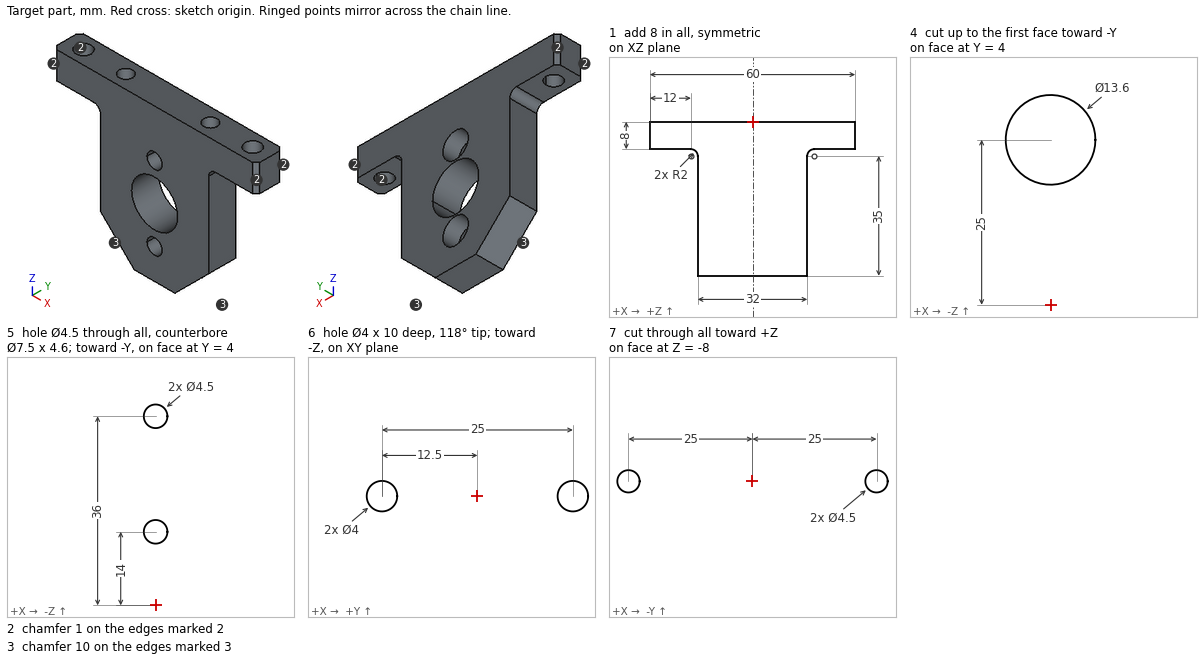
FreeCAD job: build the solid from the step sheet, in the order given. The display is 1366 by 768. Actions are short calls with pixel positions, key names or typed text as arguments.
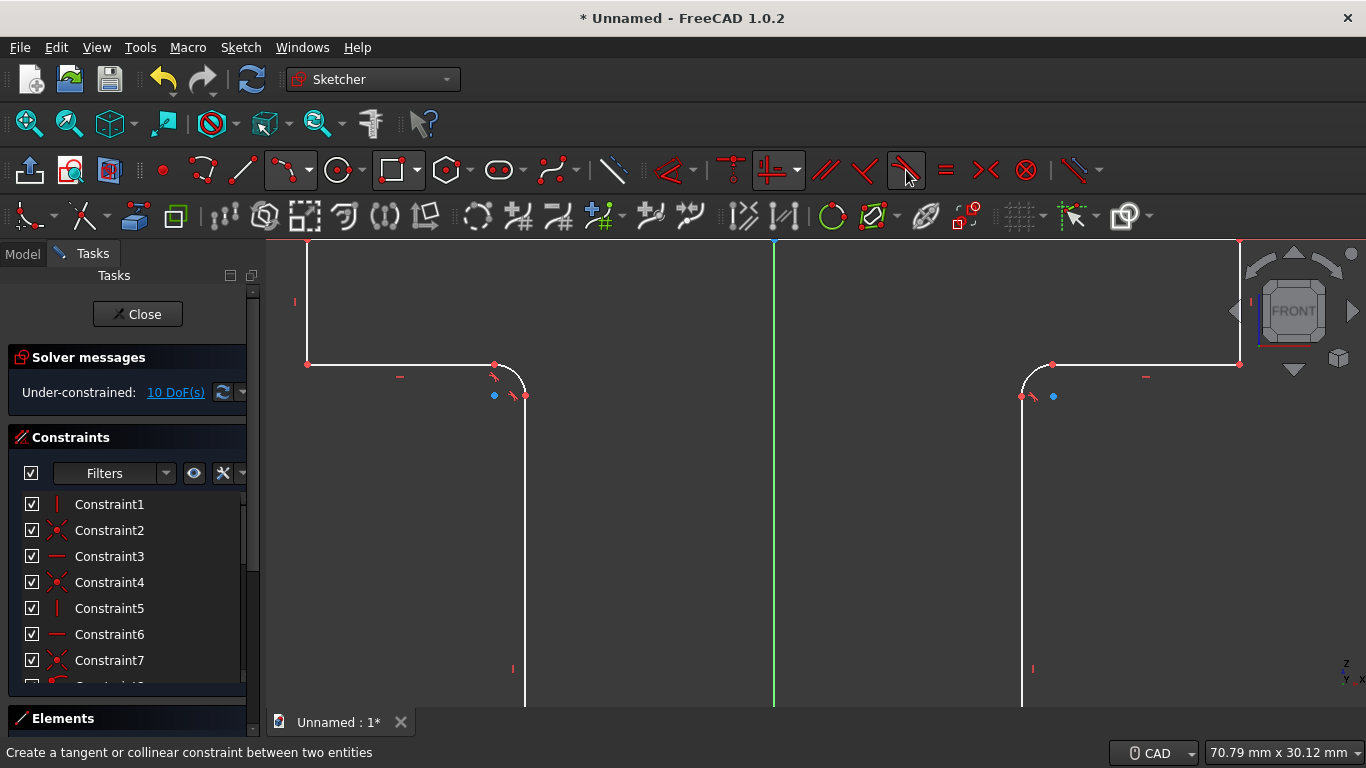
click(1184, 365)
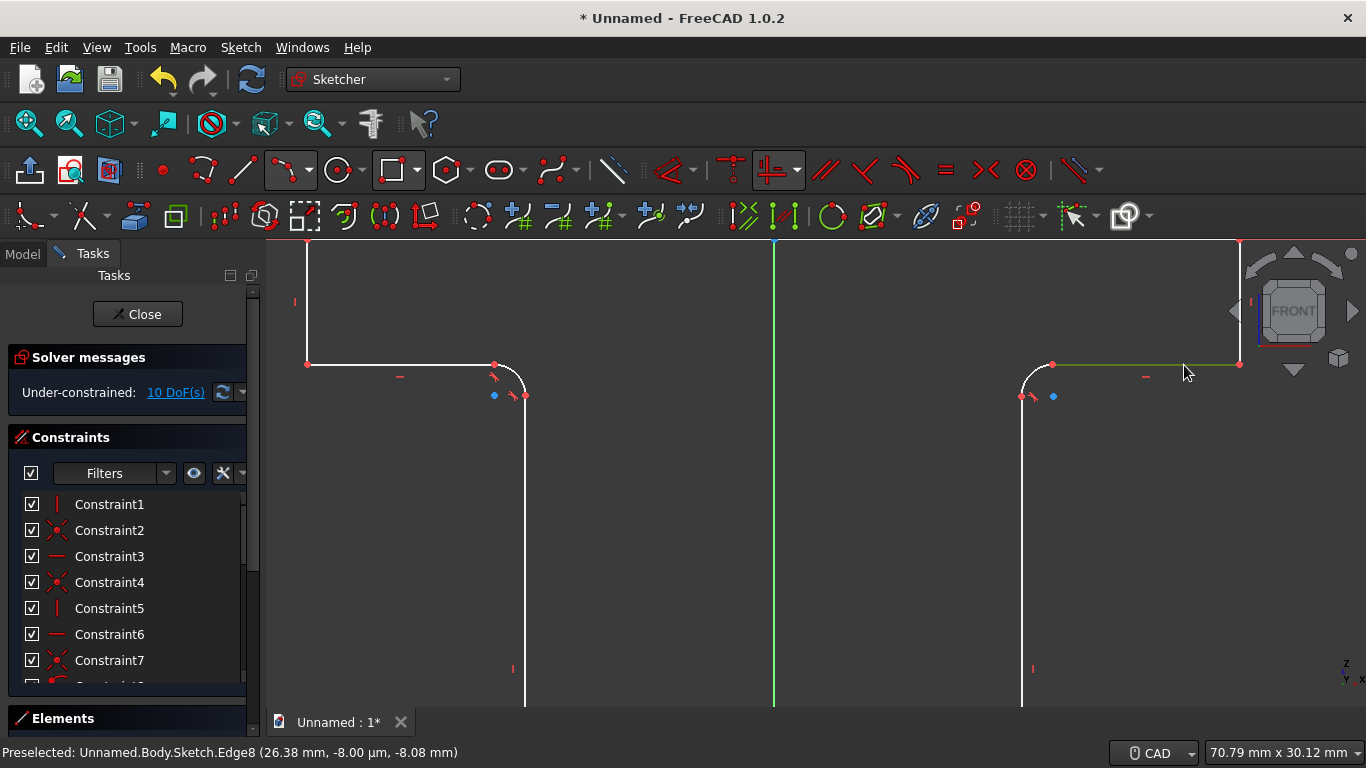
click(1039, 368)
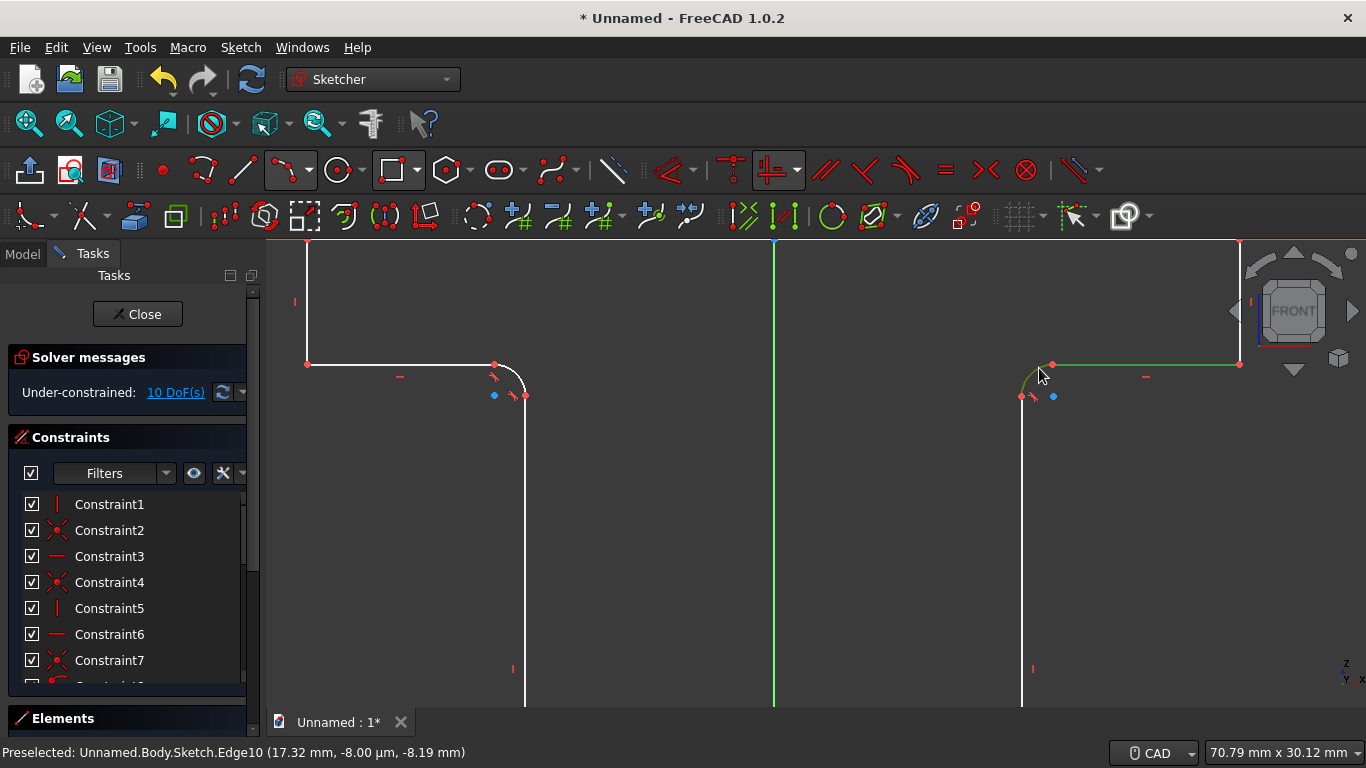
click(906, 170)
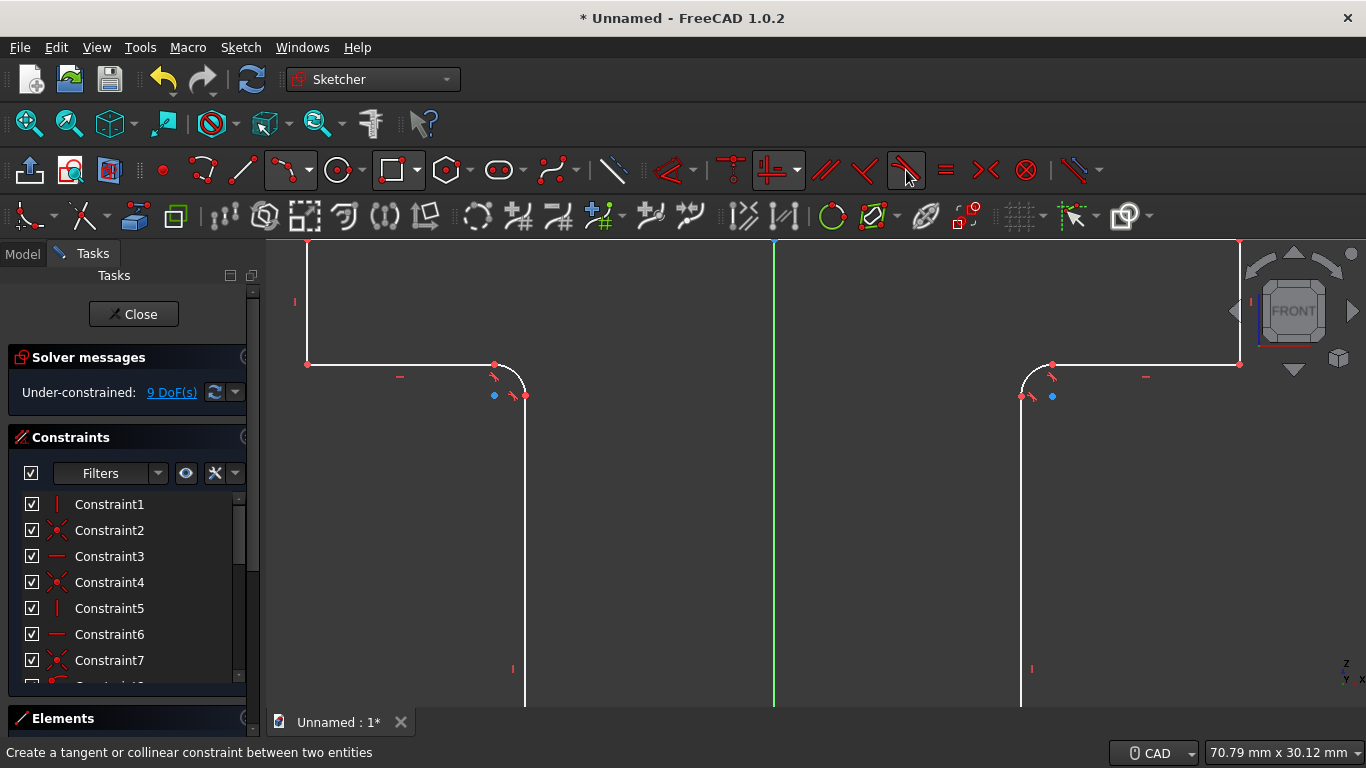
click(522, 382)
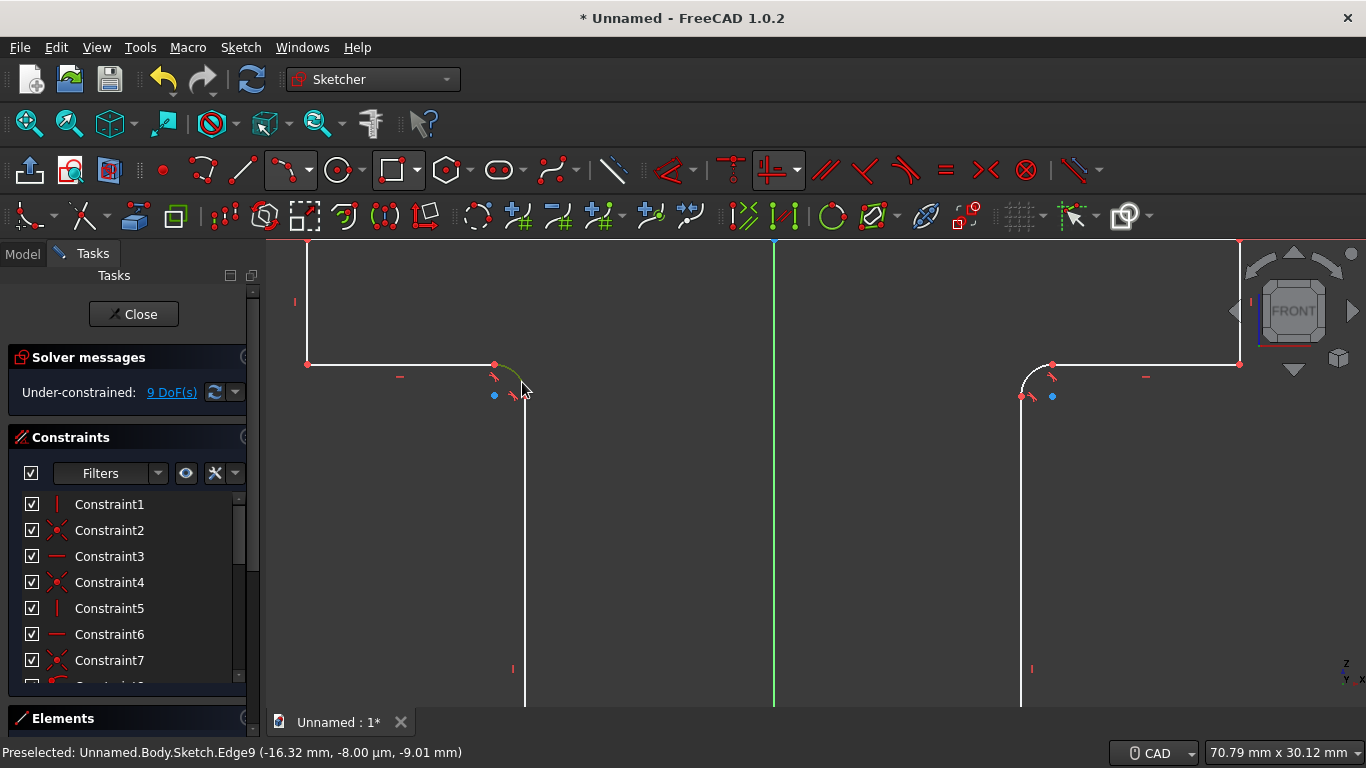
click(1038, 368)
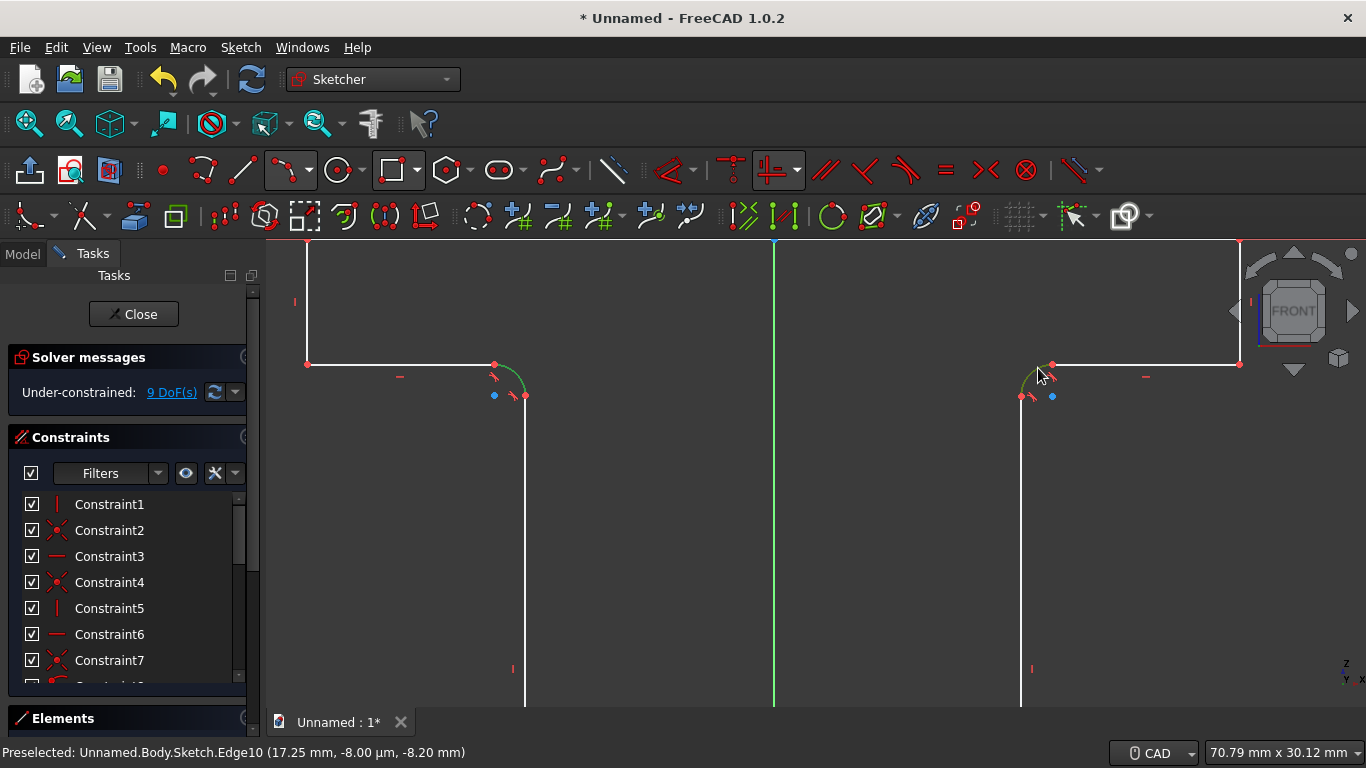
click(946, 170)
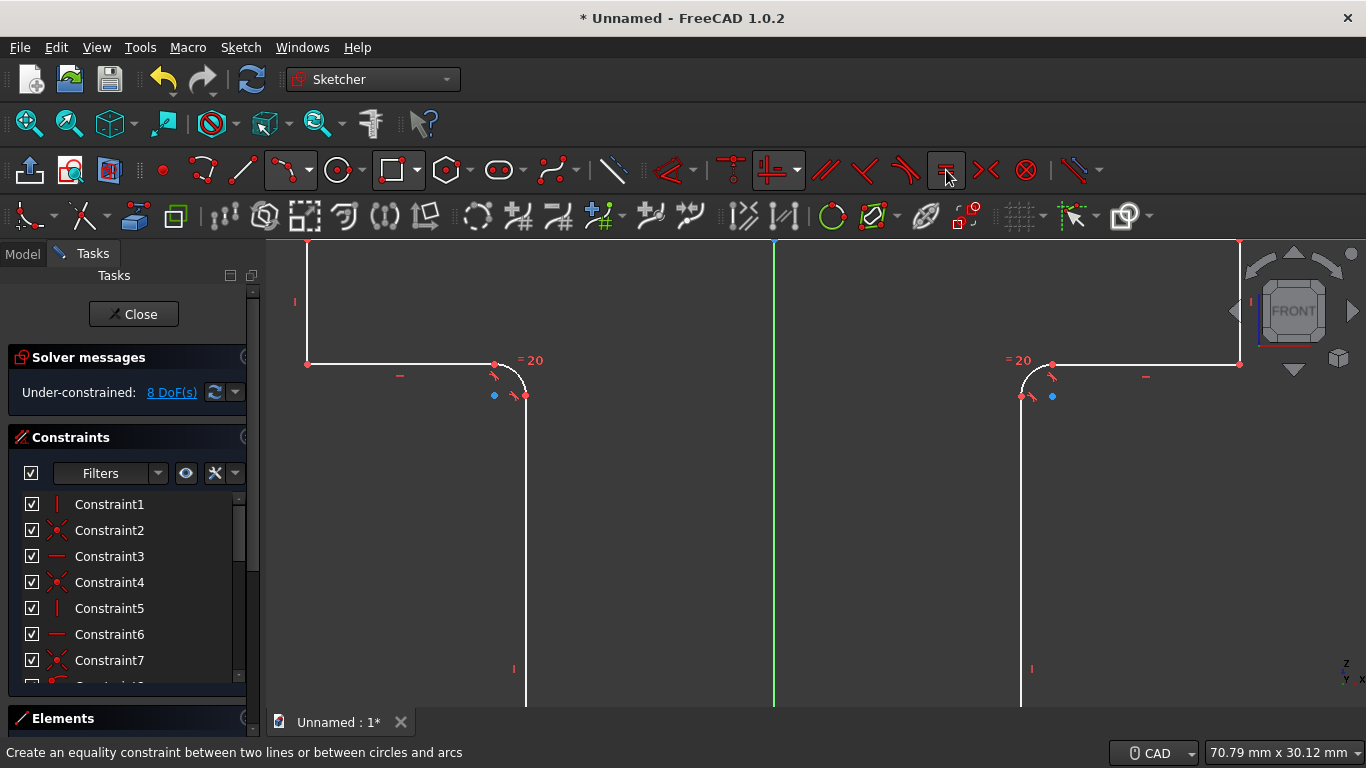
click(494, 396)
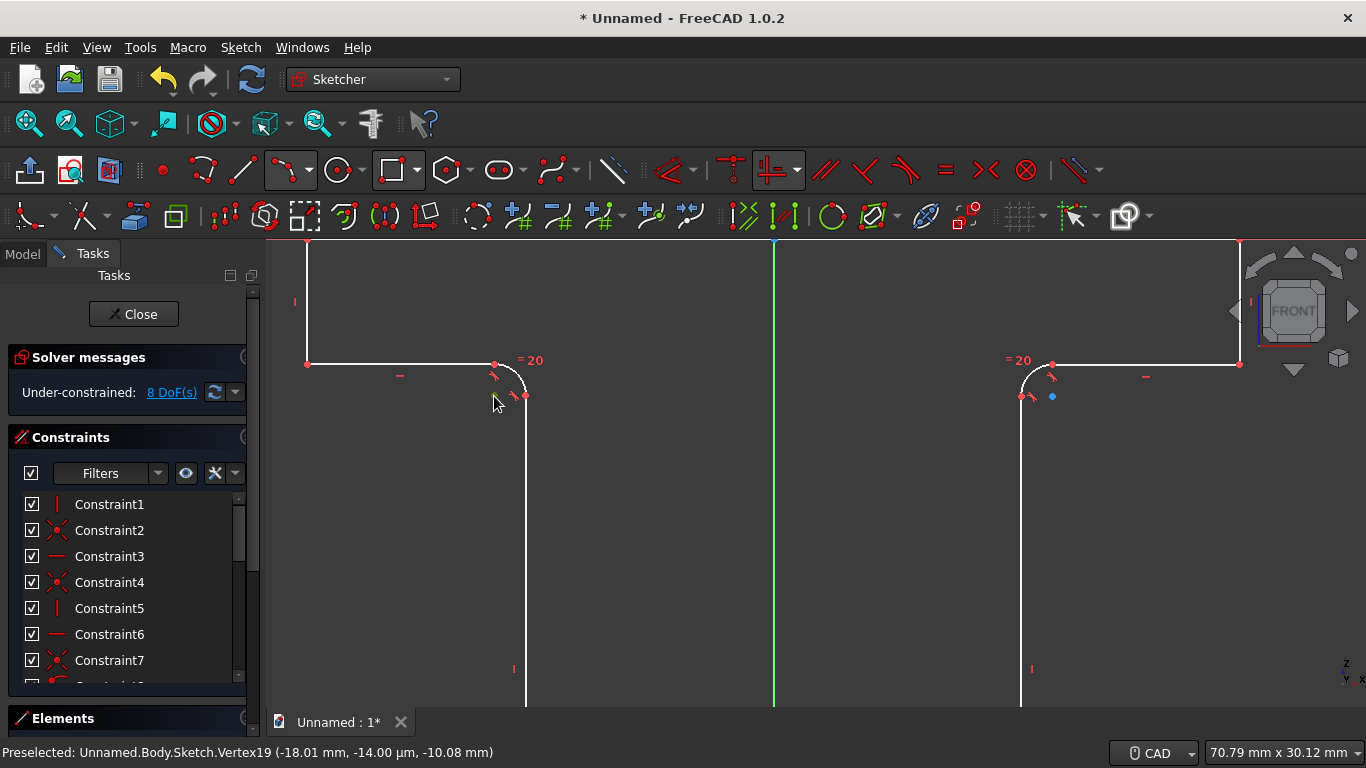
click(1053, 396)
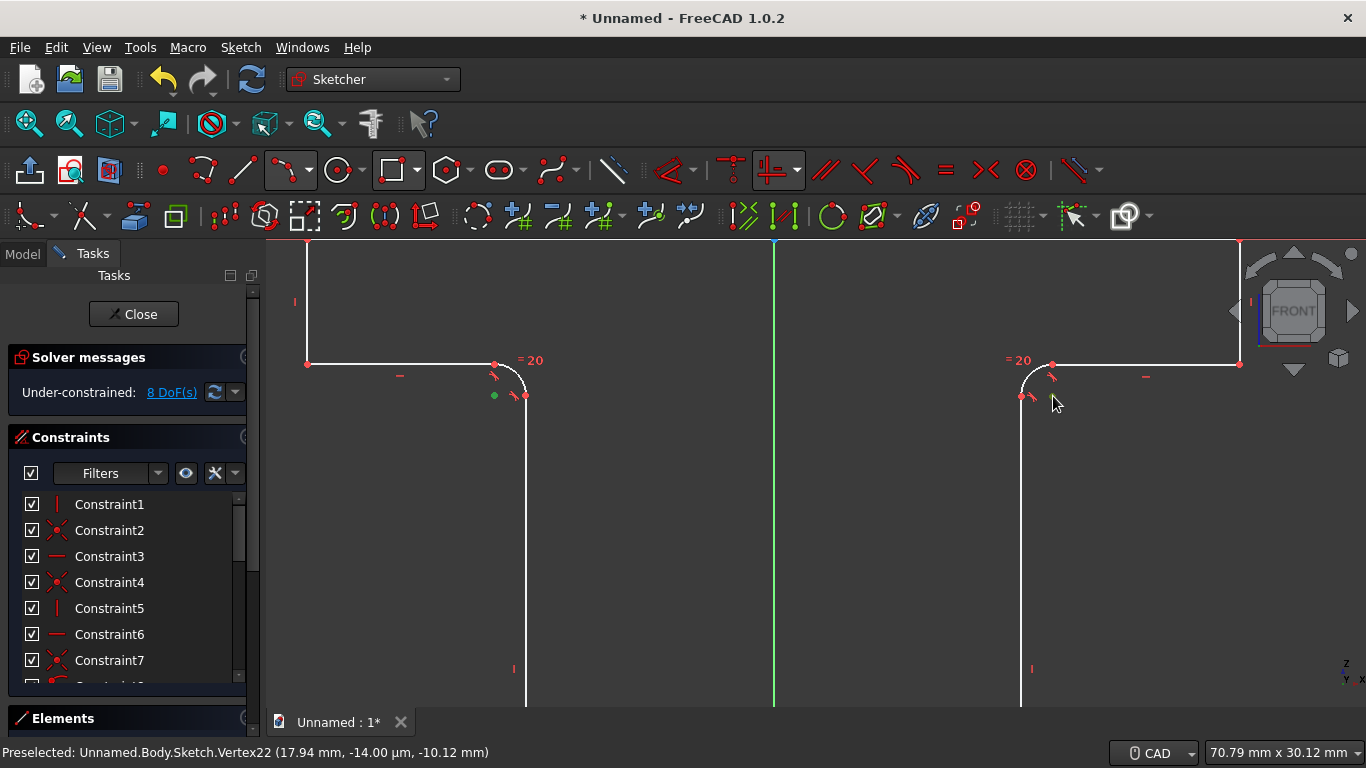
click(774, 650)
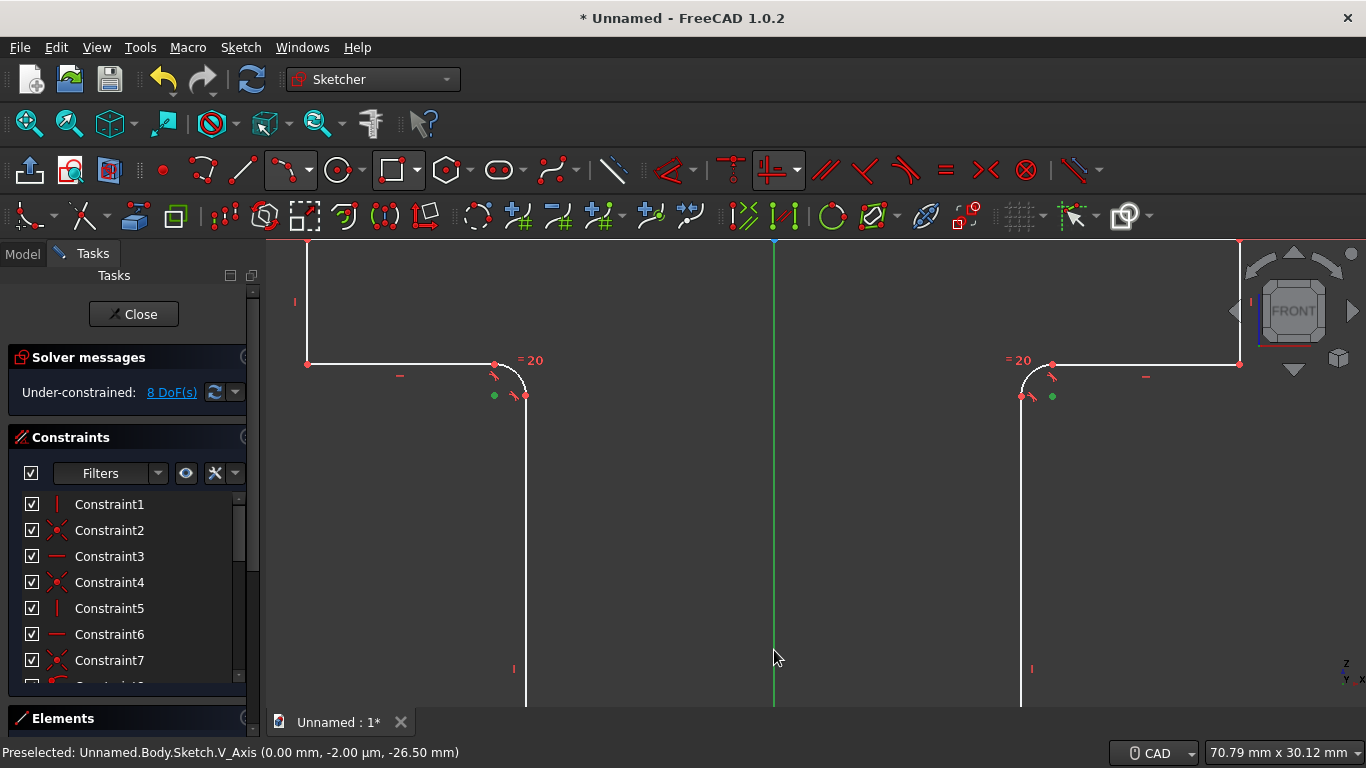
click(986, 170)